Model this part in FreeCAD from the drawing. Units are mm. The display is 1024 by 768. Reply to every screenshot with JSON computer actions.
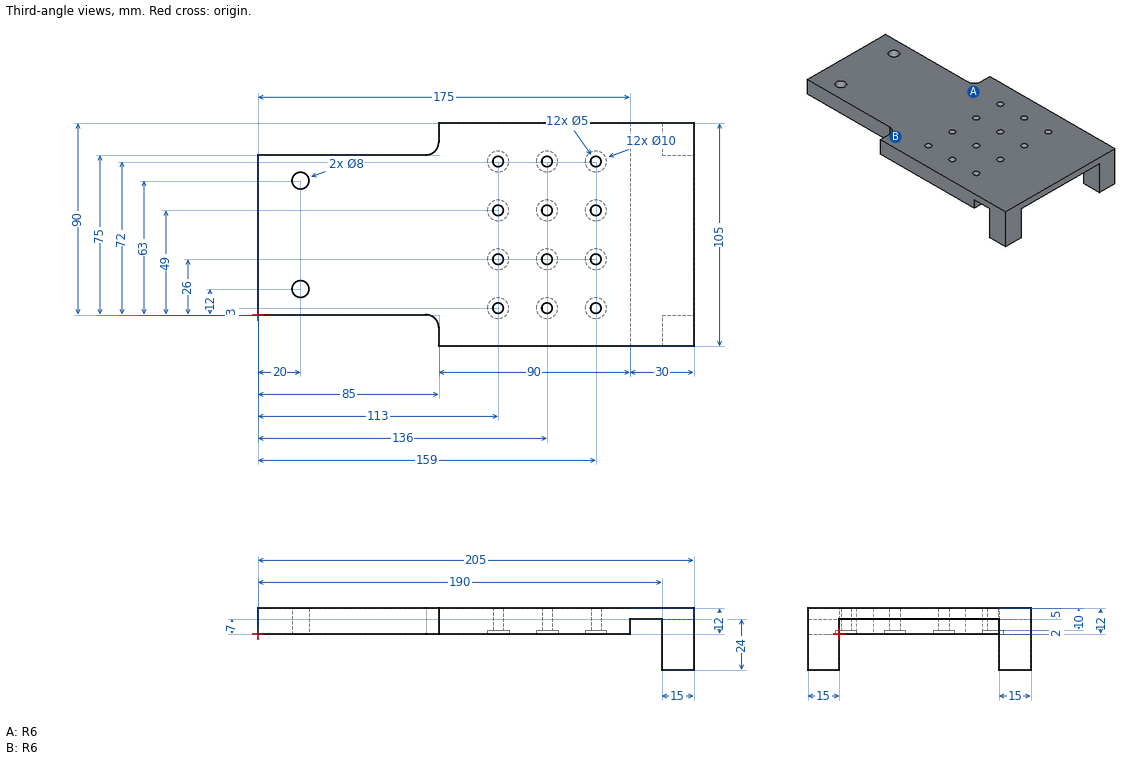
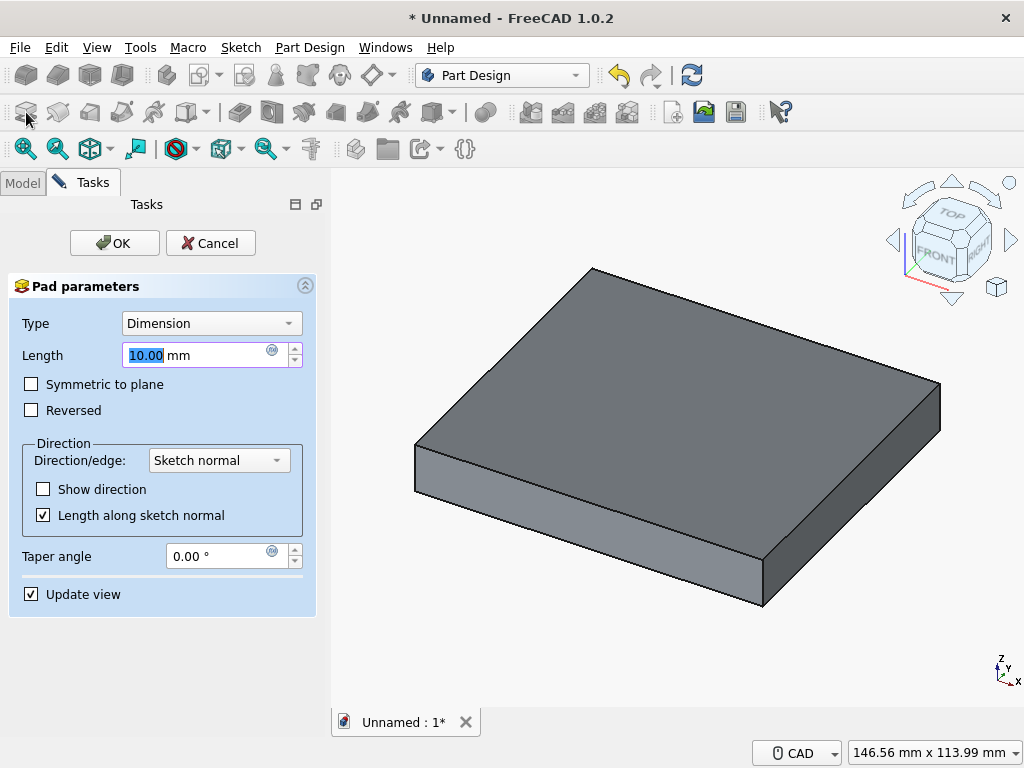
{"action": "type", "text": "12"}
{"action": "key", "text": "Tab"}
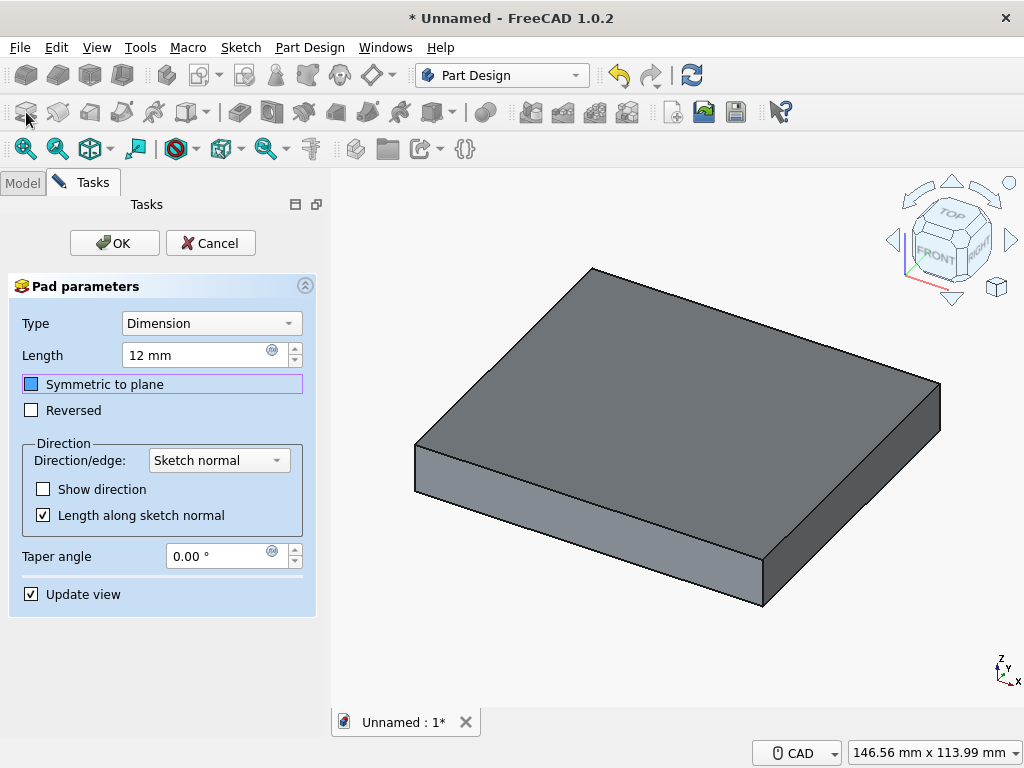
{"action": "left_click", "coordinate": [30, 410]}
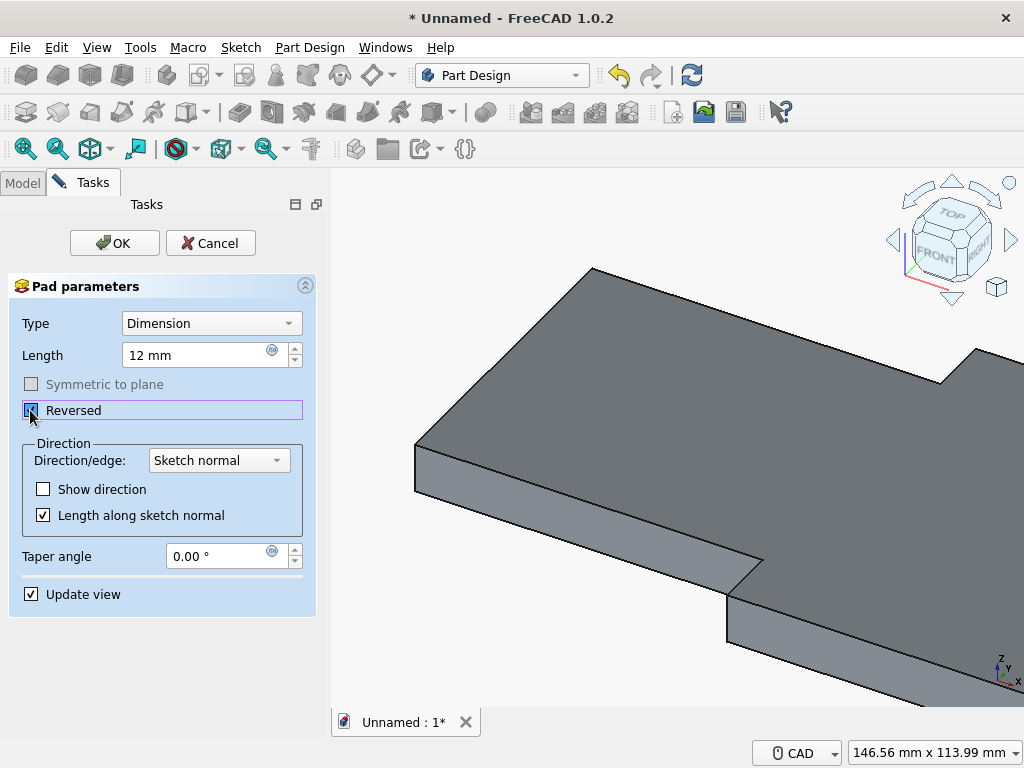
{"action": "left_click", "coordinate": [115, 243]}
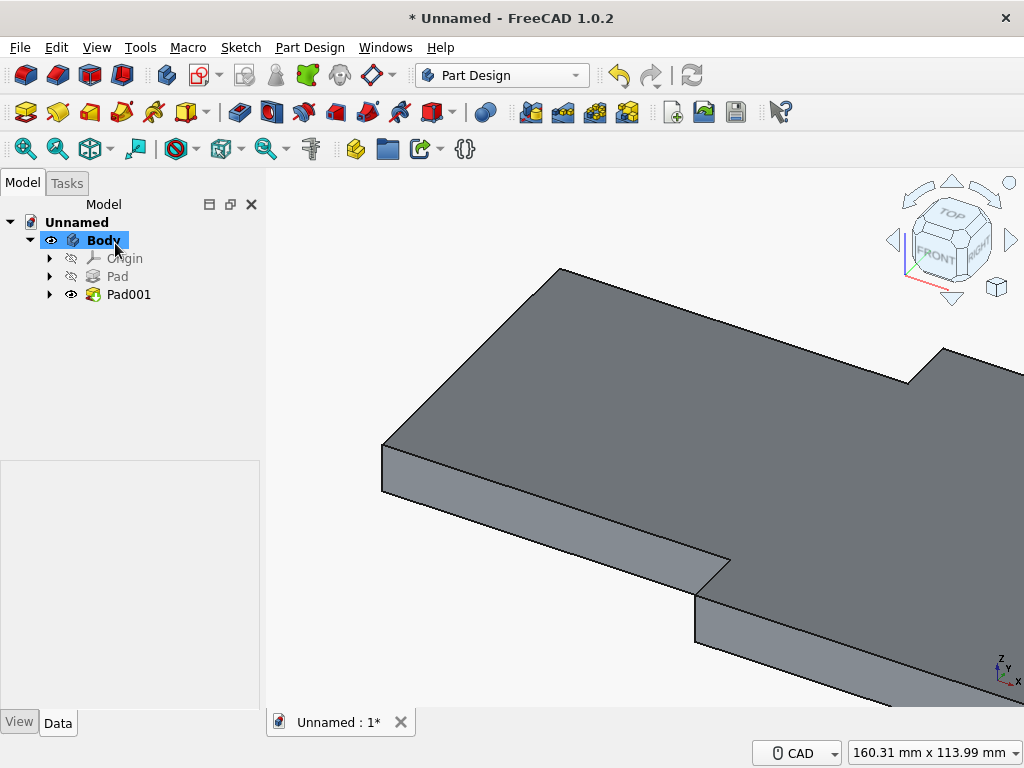
{"action": "left_click", "coordinate": [26, 150]}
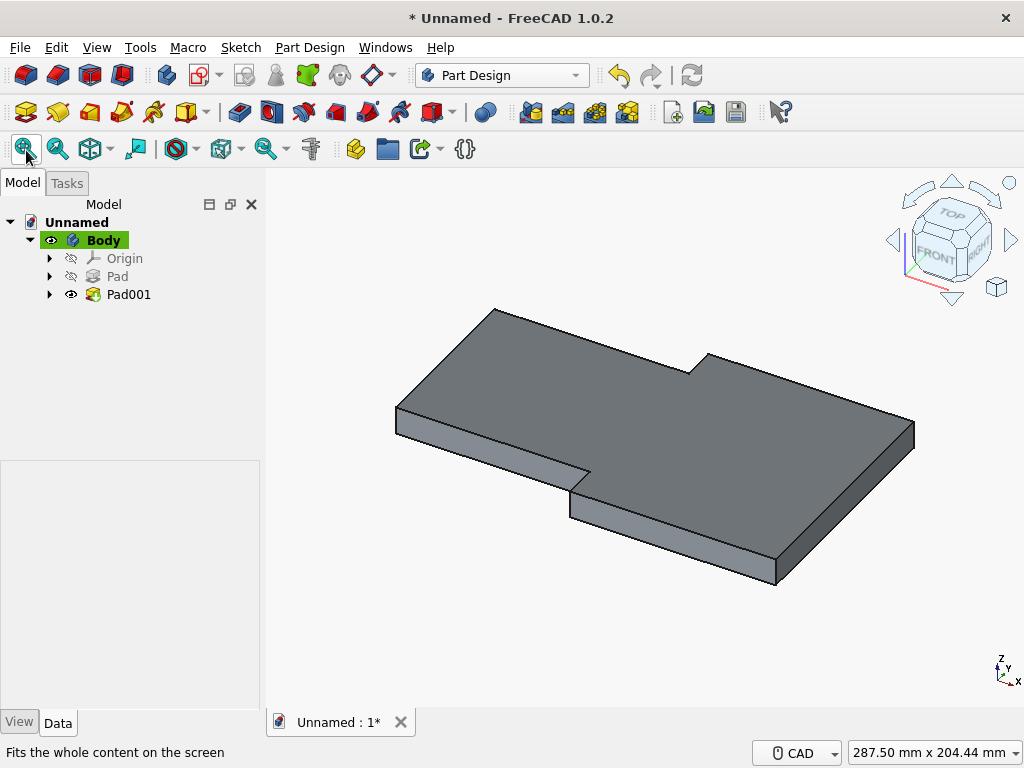
{"action": "key", "text": "0"}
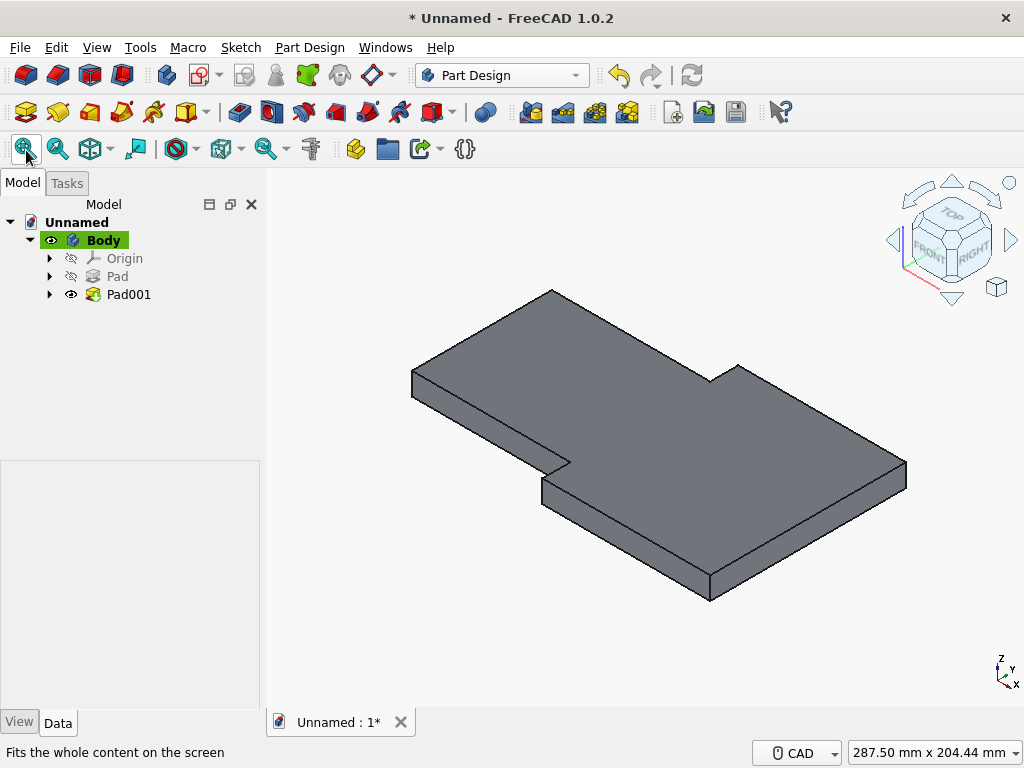
{"action": "key", "text": "2"}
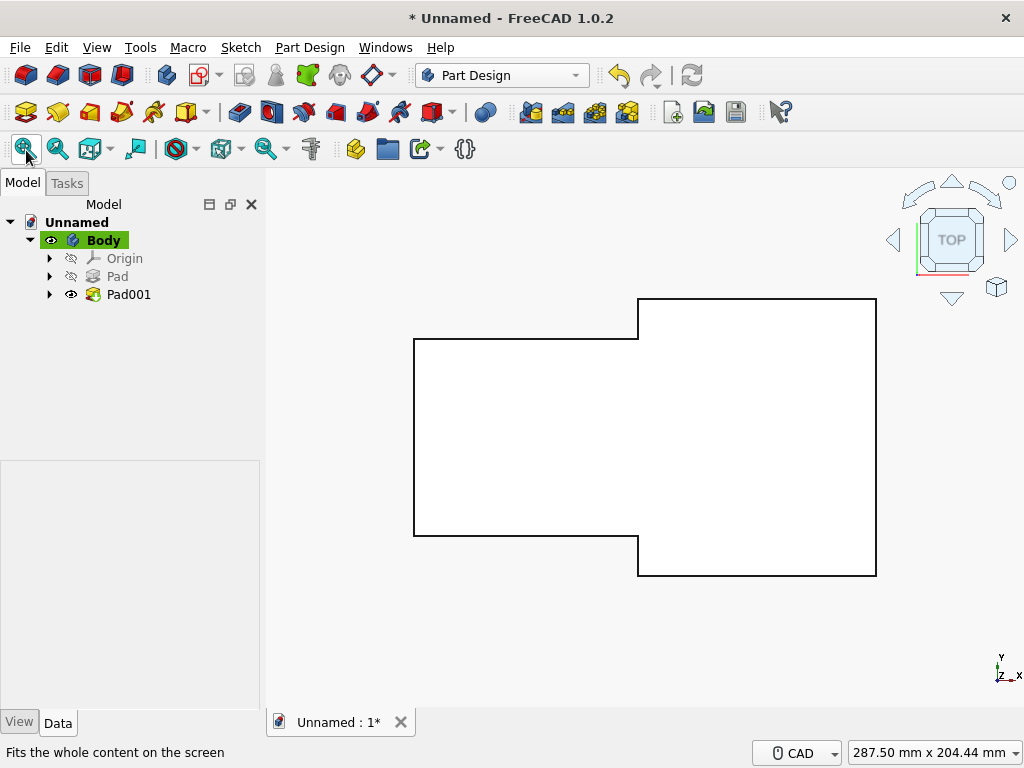
{"action": "key", "text": "1"}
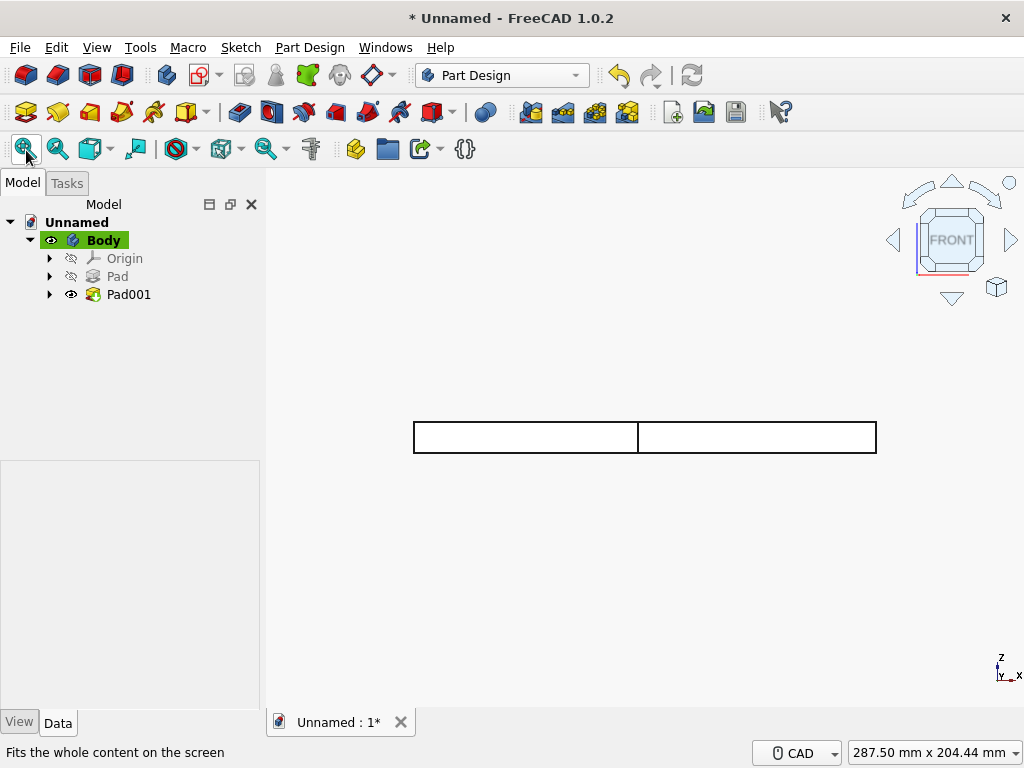
{"action": "key", "text": "3"}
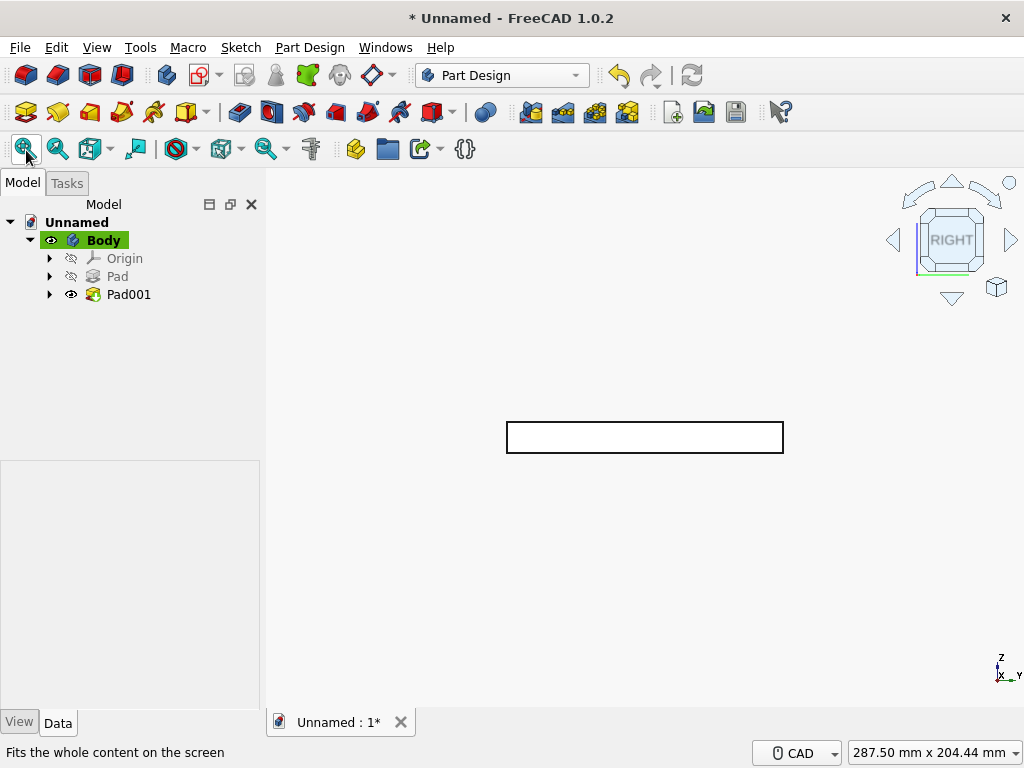
{"action": "left_click", "coordinate": [26, 150]}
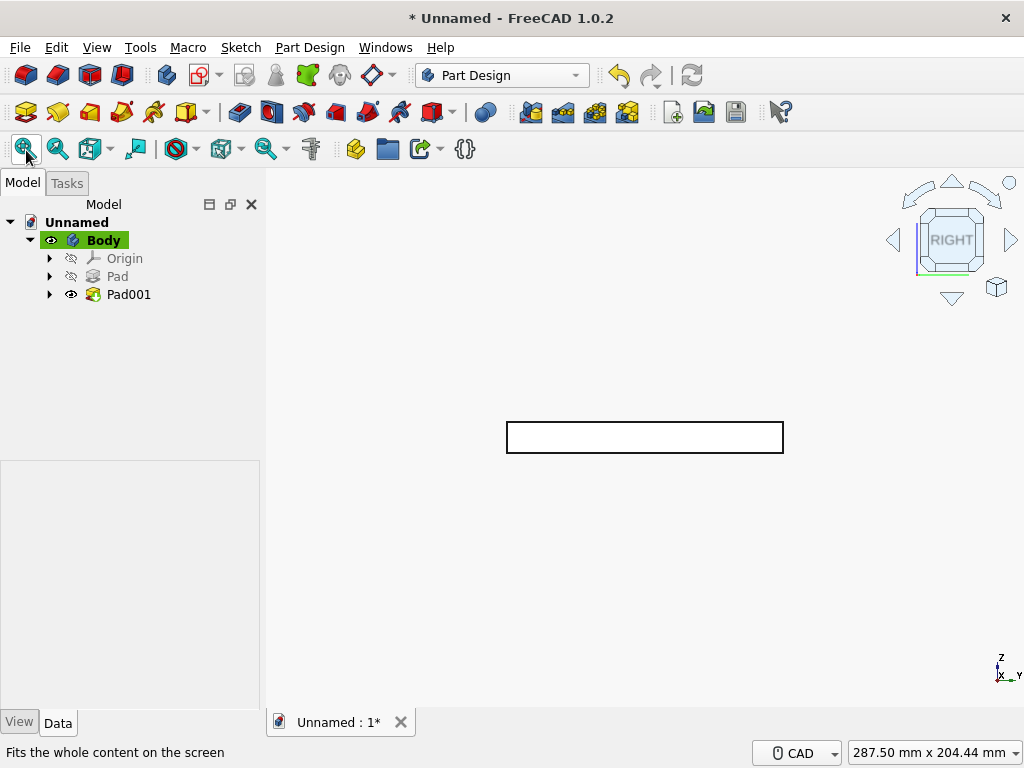
{"action": "key", "text": "5"}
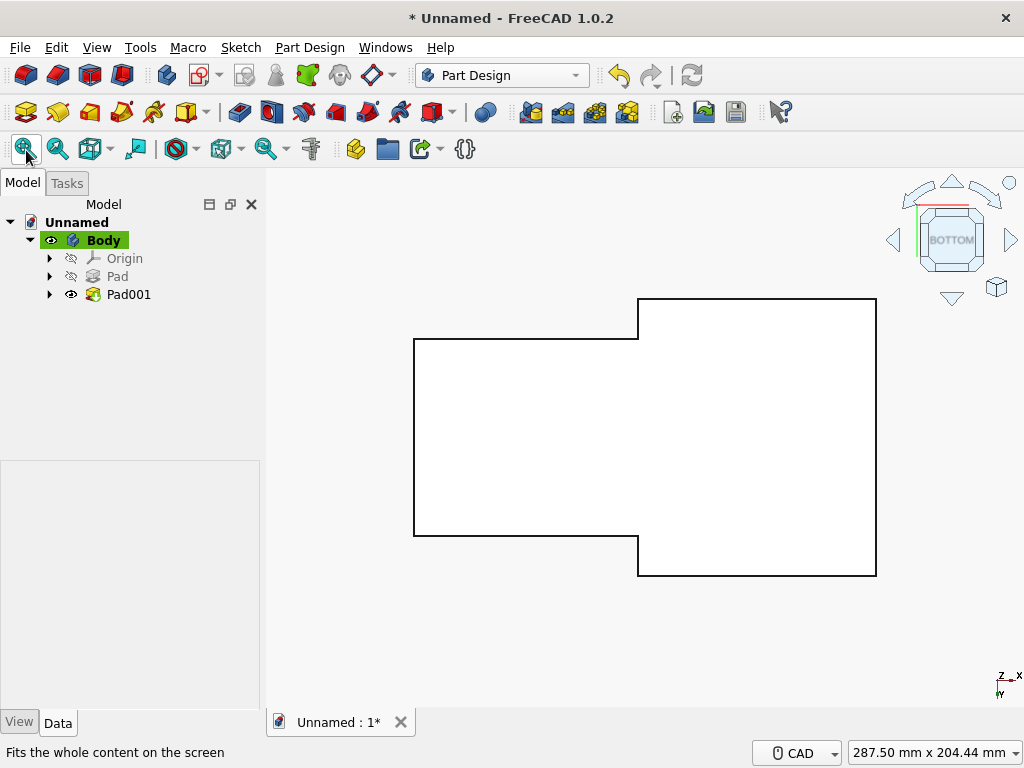
{"action": "key", "text": "4"}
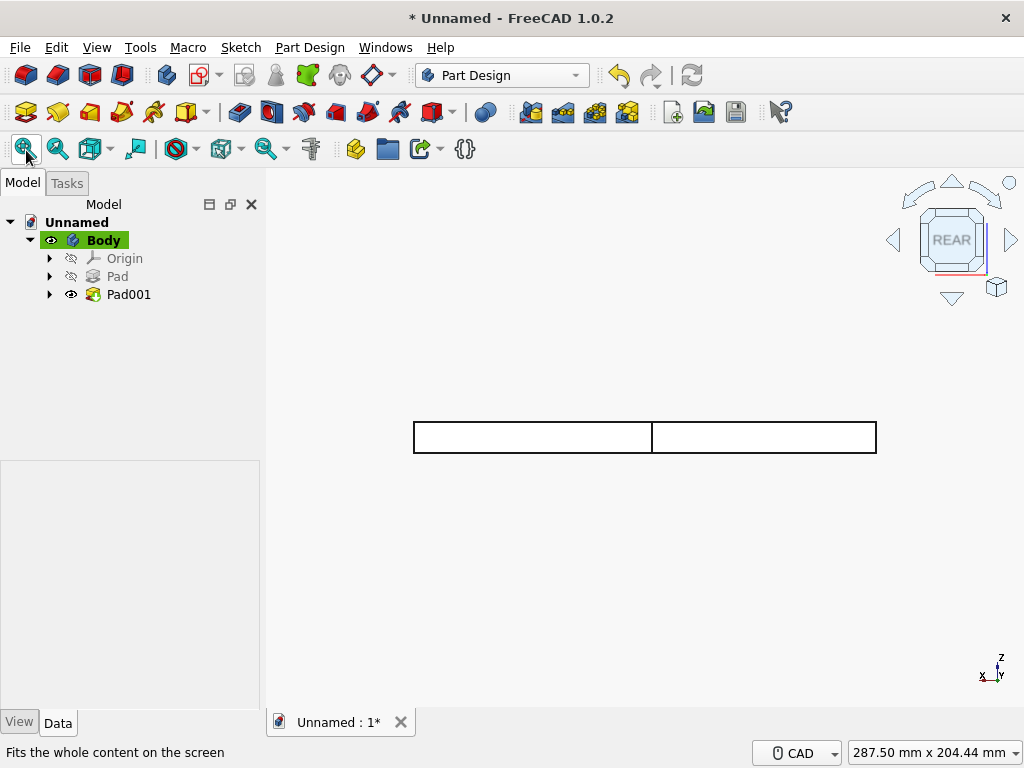
{"action": "key", "text": "6"}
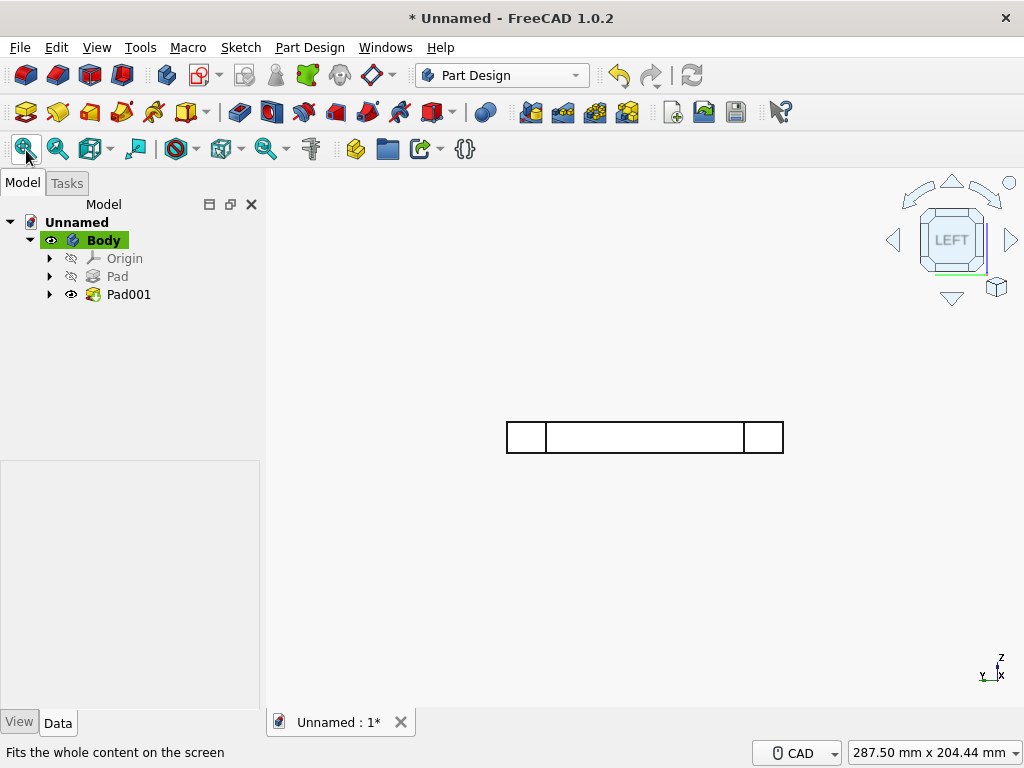
{"action": "left_click", "coordinate": [26, 150]}